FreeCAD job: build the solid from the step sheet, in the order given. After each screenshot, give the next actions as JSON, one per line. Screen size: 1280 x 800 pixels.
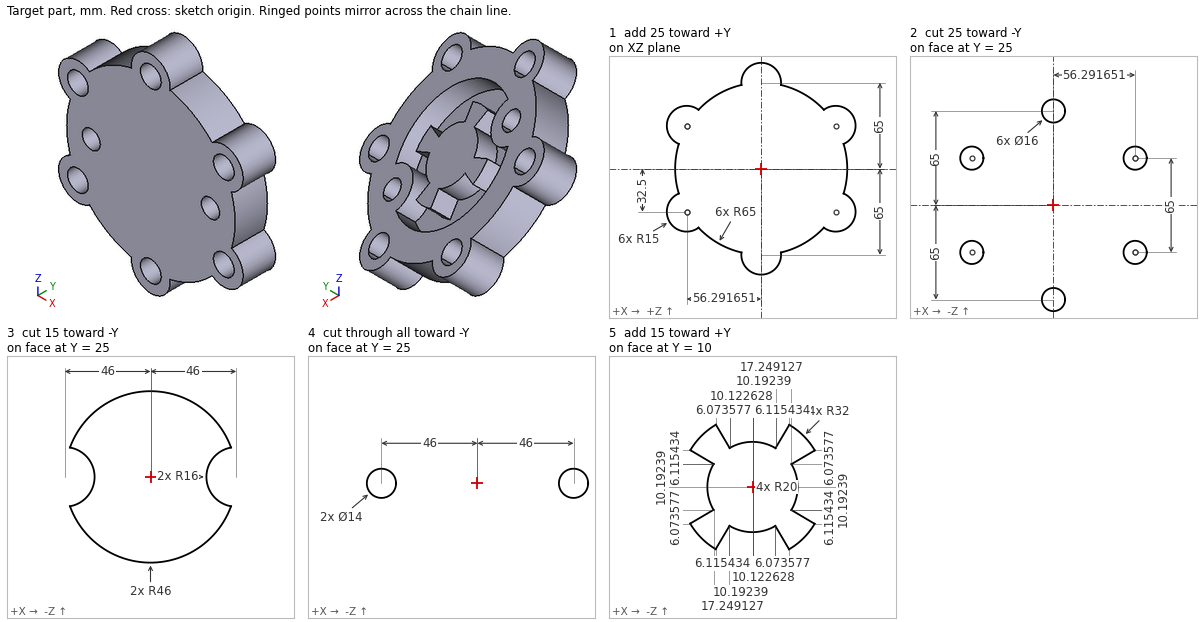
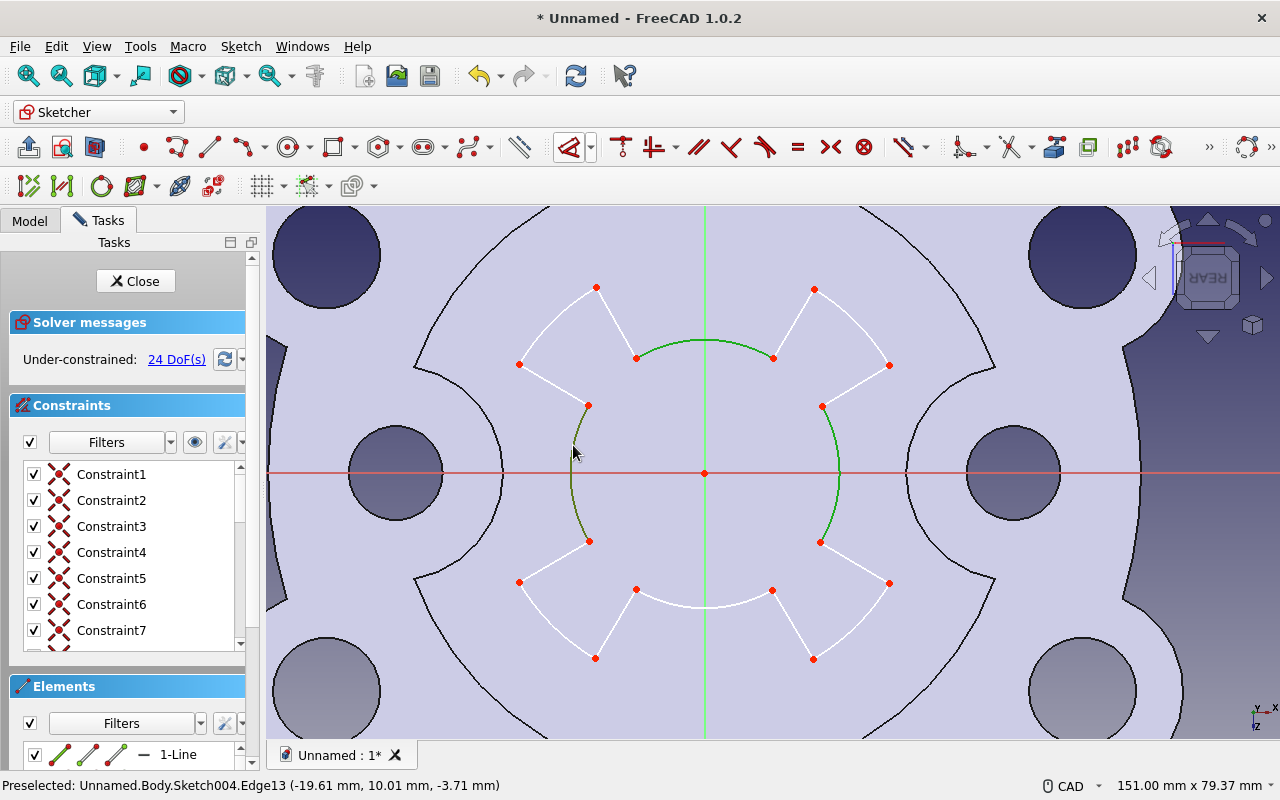
{"action": "left_click", "coordinate": [676, 605]}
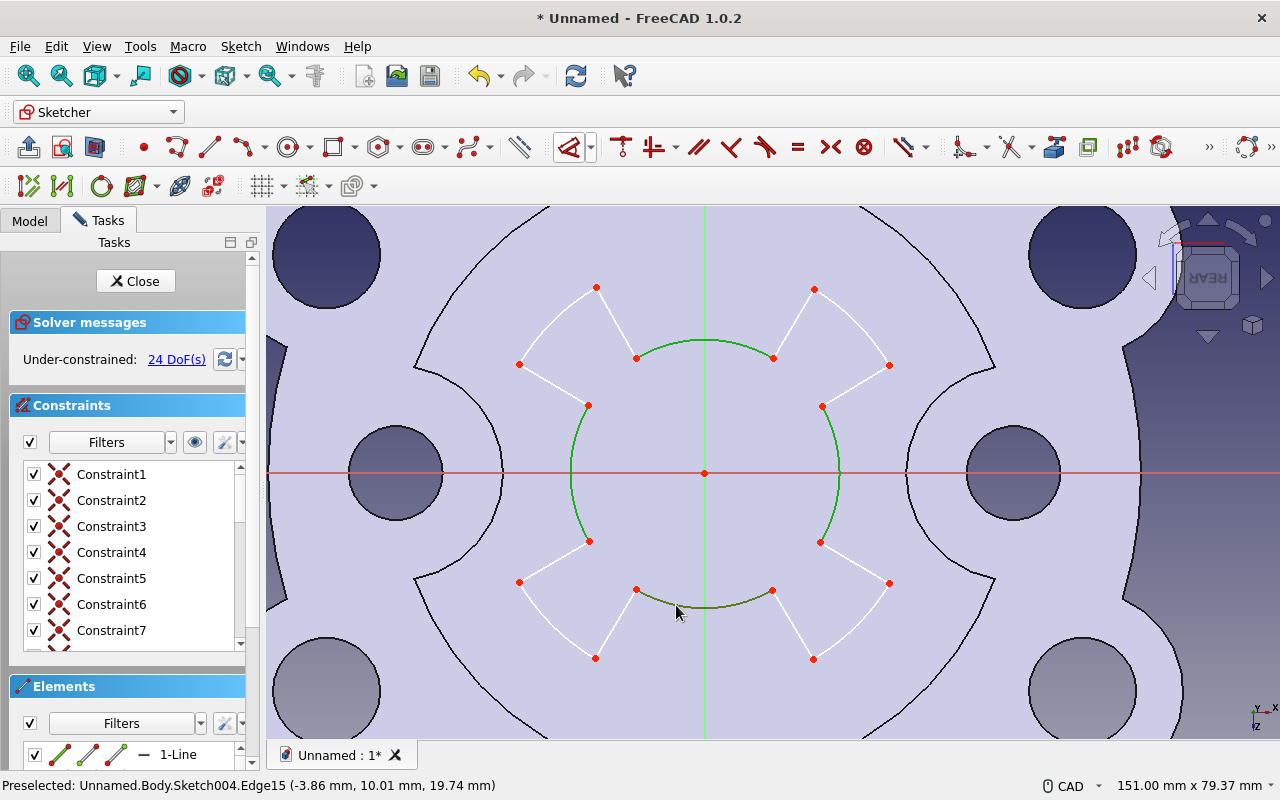
{"action": "key", "text": "e"}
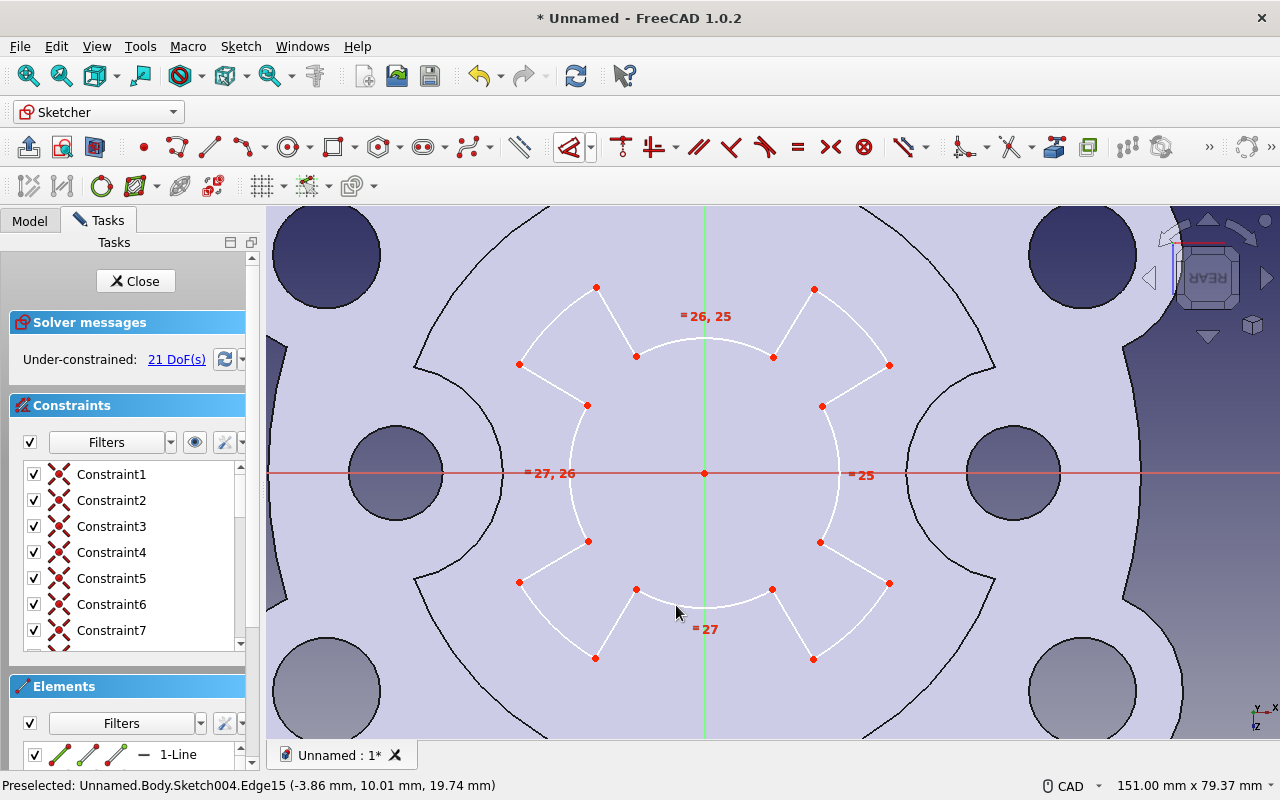
{"action": "left_click", "coordinate": [871, 339]}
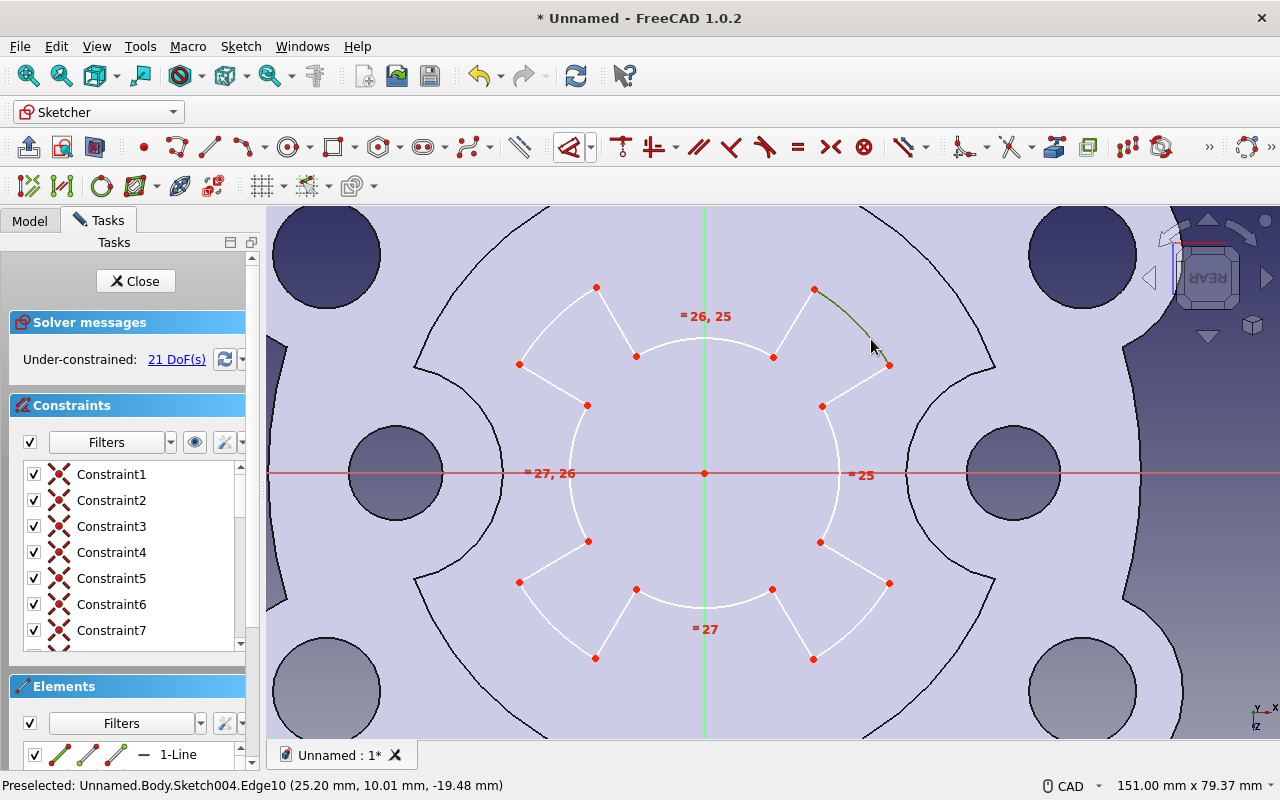
{"action": "left_click", "coordinate": [569, 307]}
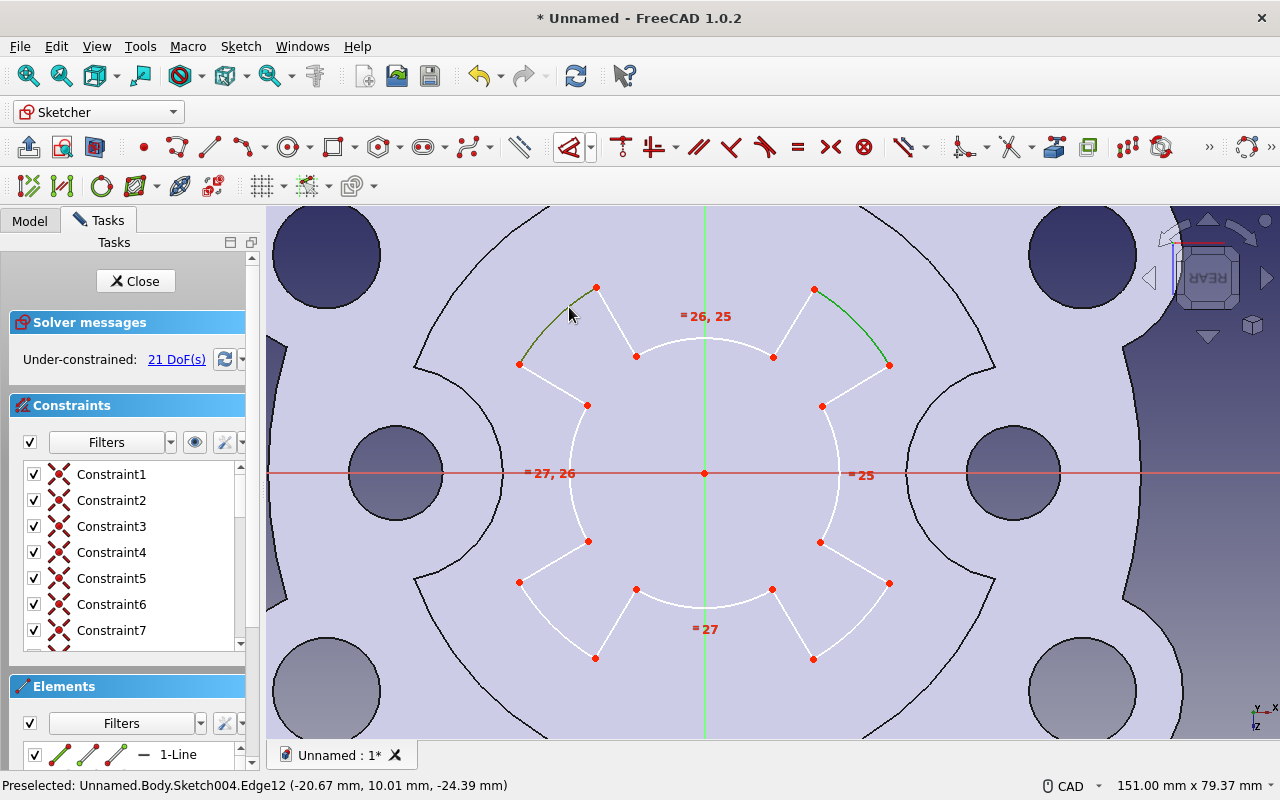
{"action": "left_click", "coordinate": [538, 609]}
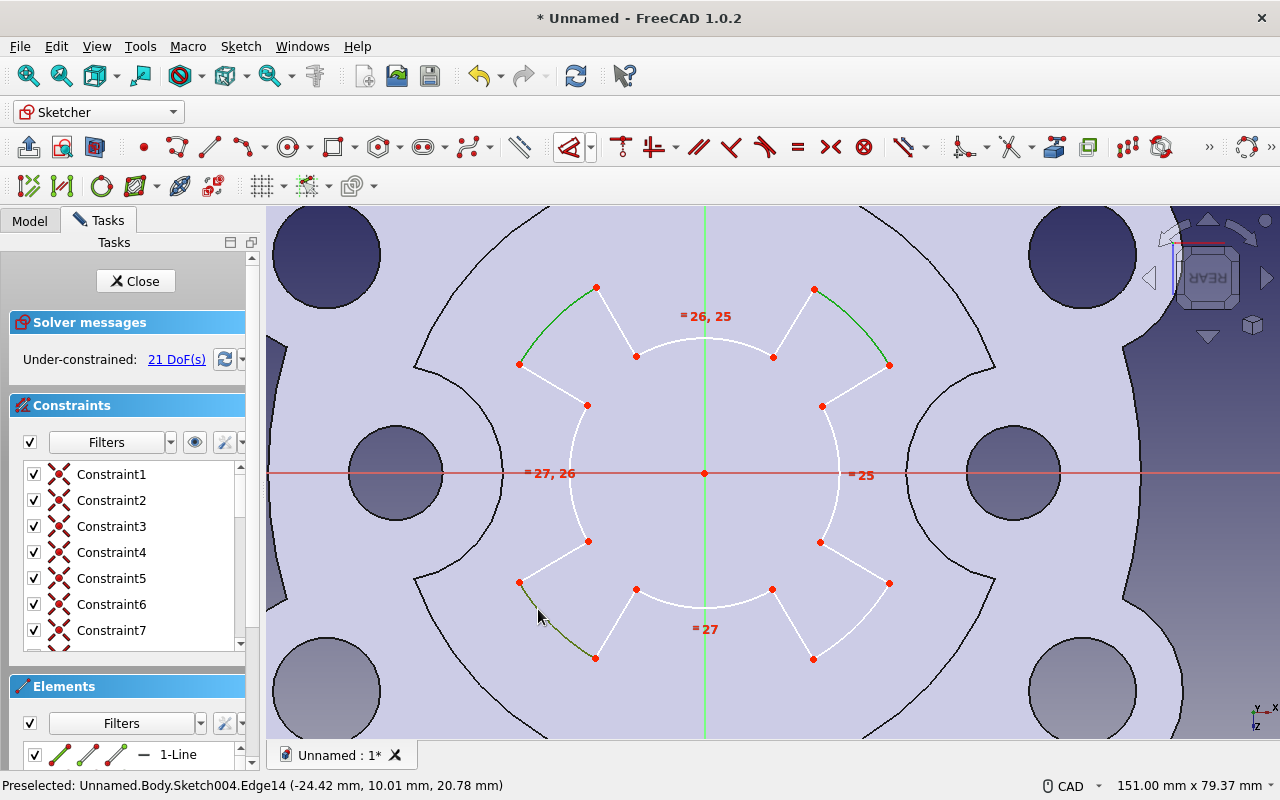
{"action": "left_click", "coordinate": [840, 641]}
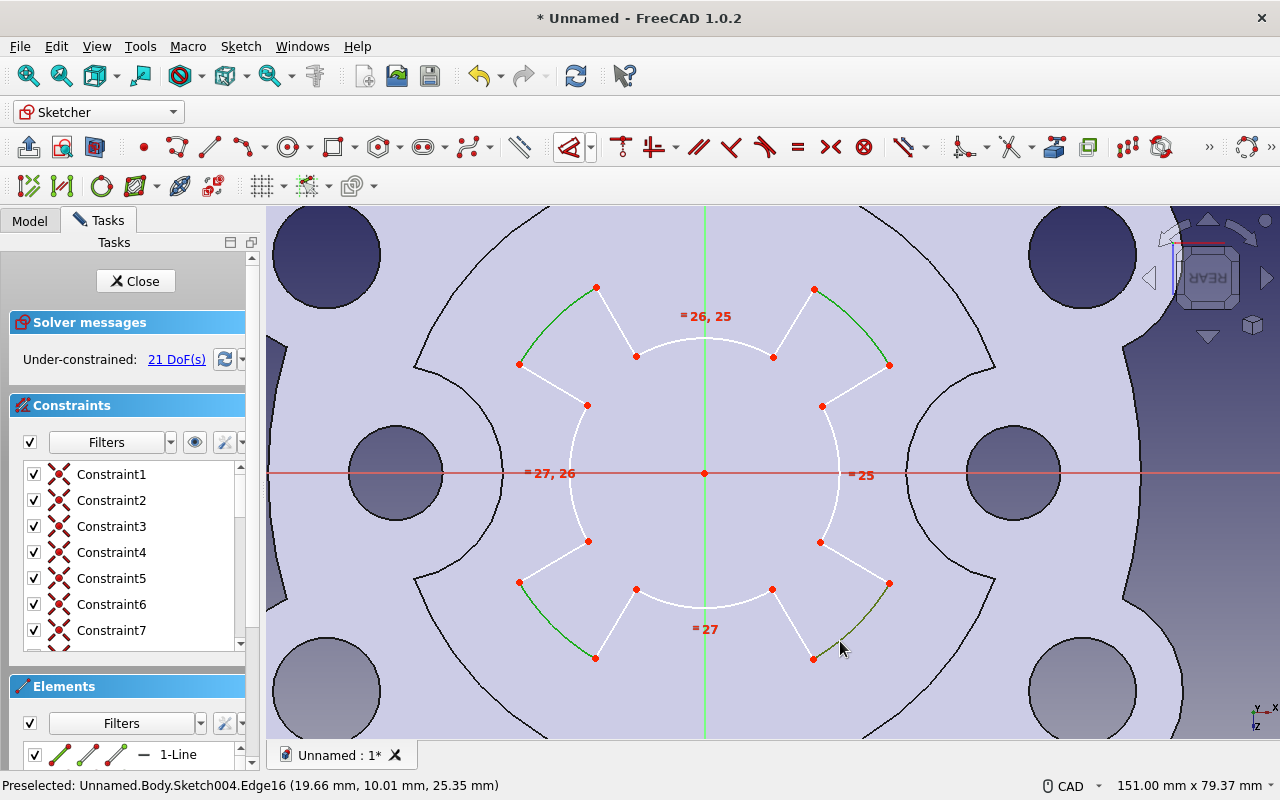
{"action": "left_click", "coordinate": [798, 148]}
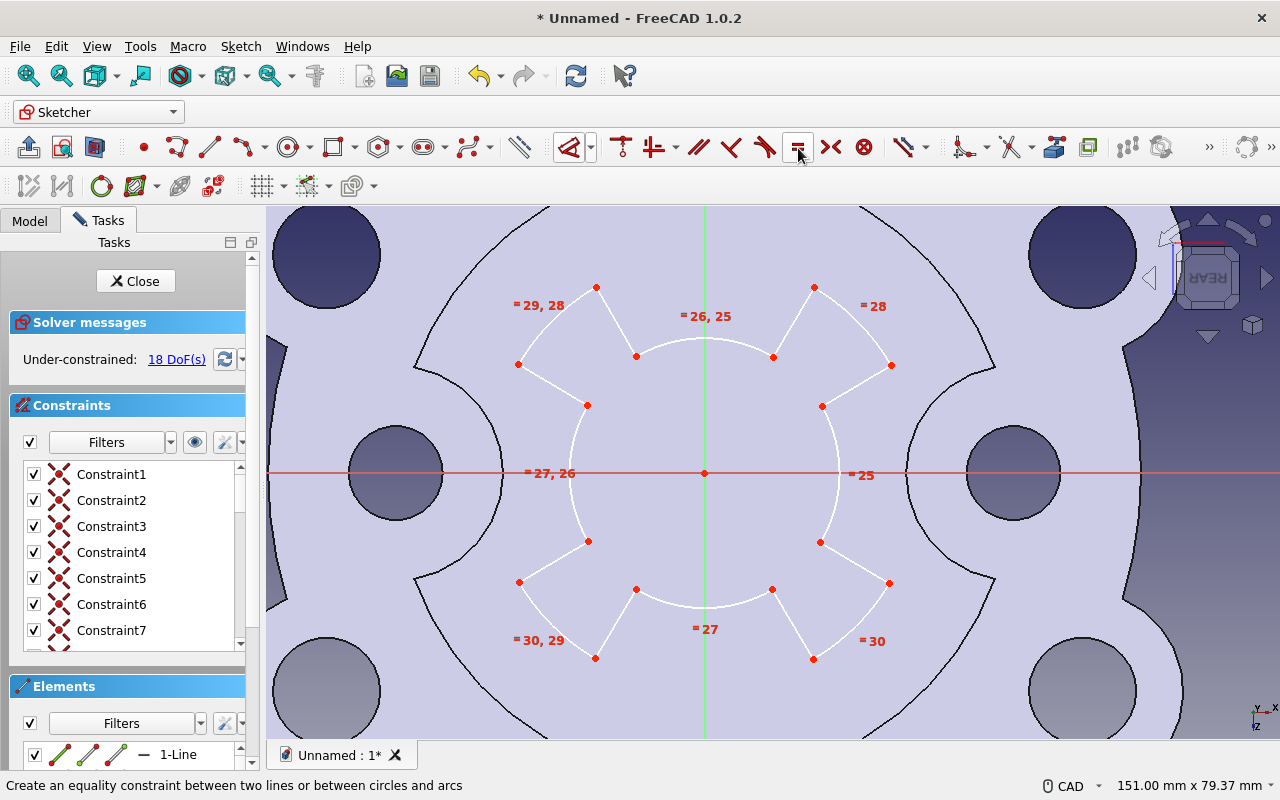
{"action": "left_click", "coordinate": [836, 503]}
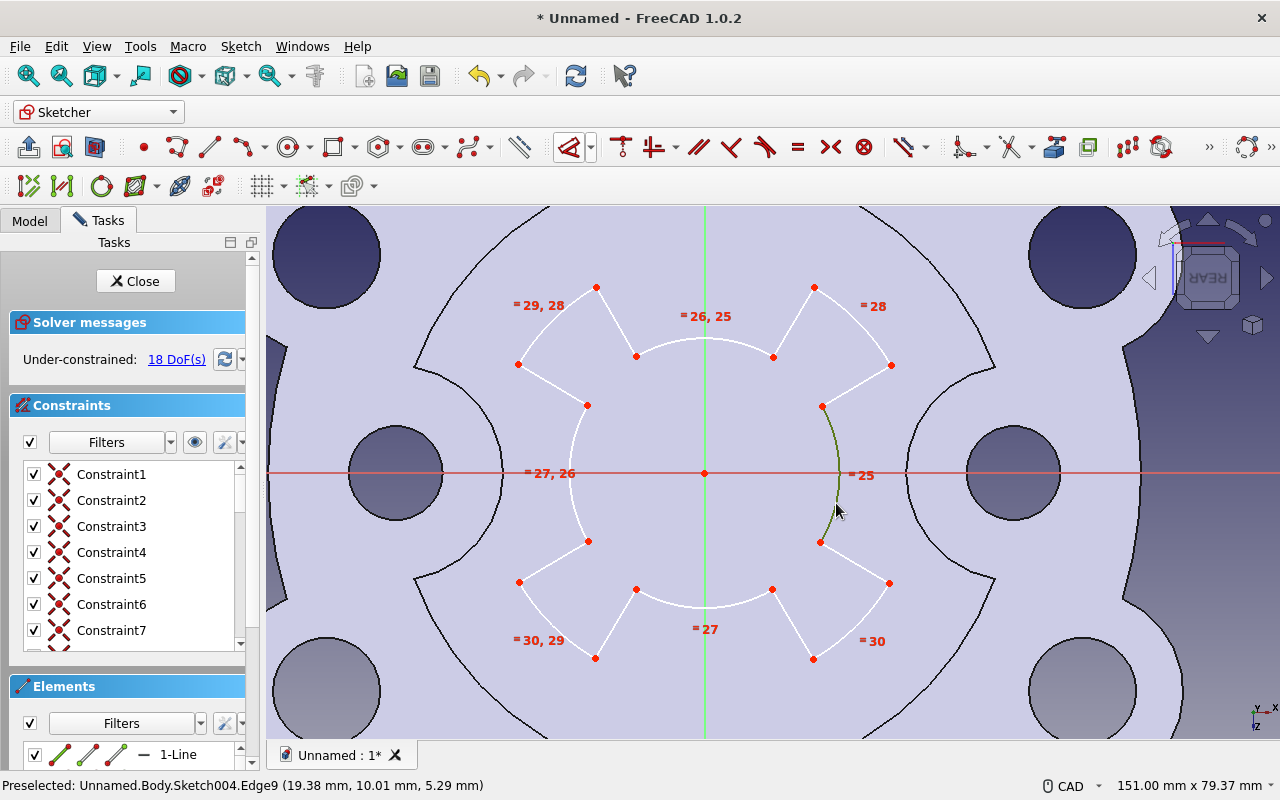
{"action": "key", "text": "k r"}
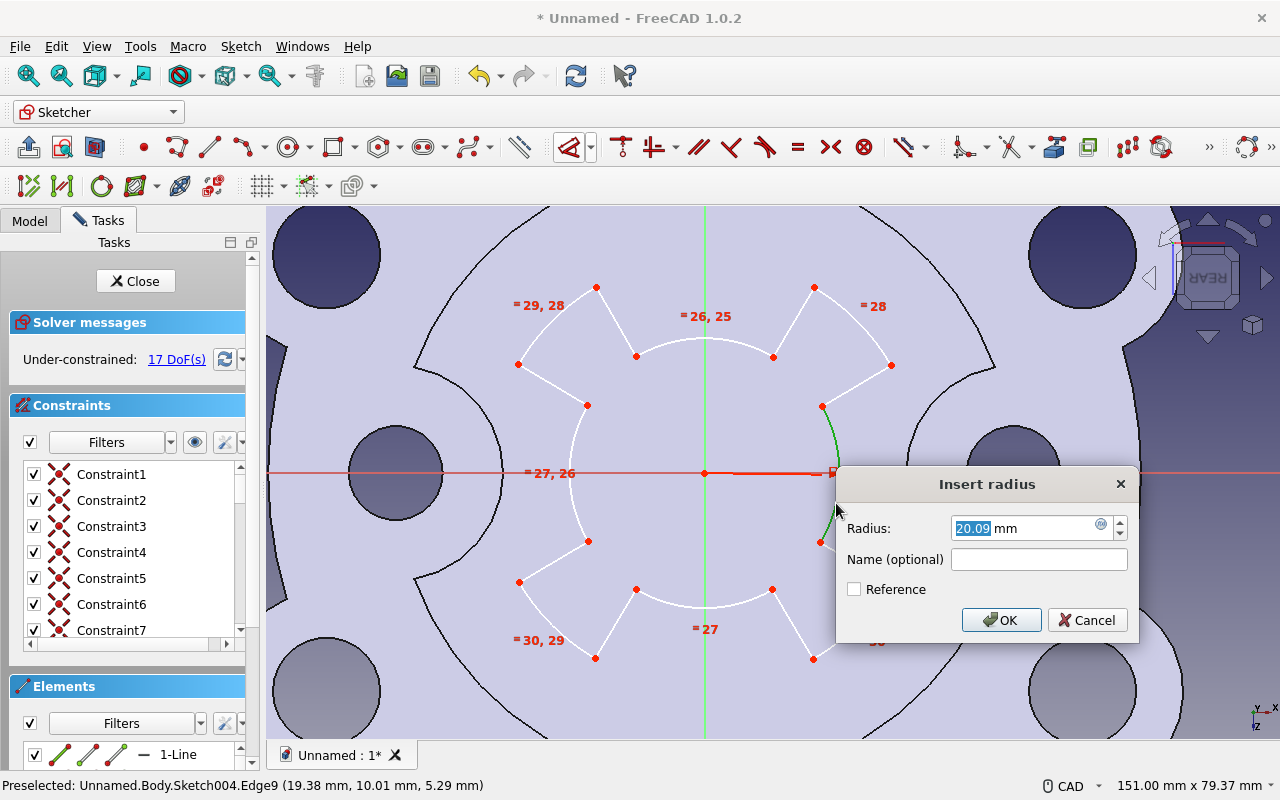
{"action": "type", "text": "20"}
{"action": "key", "text": "Return"}